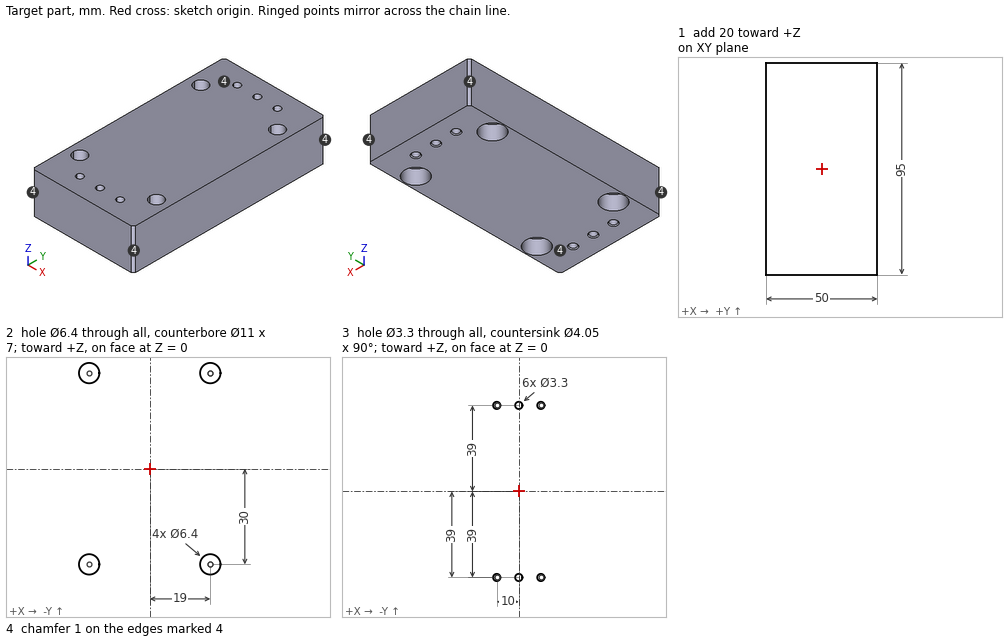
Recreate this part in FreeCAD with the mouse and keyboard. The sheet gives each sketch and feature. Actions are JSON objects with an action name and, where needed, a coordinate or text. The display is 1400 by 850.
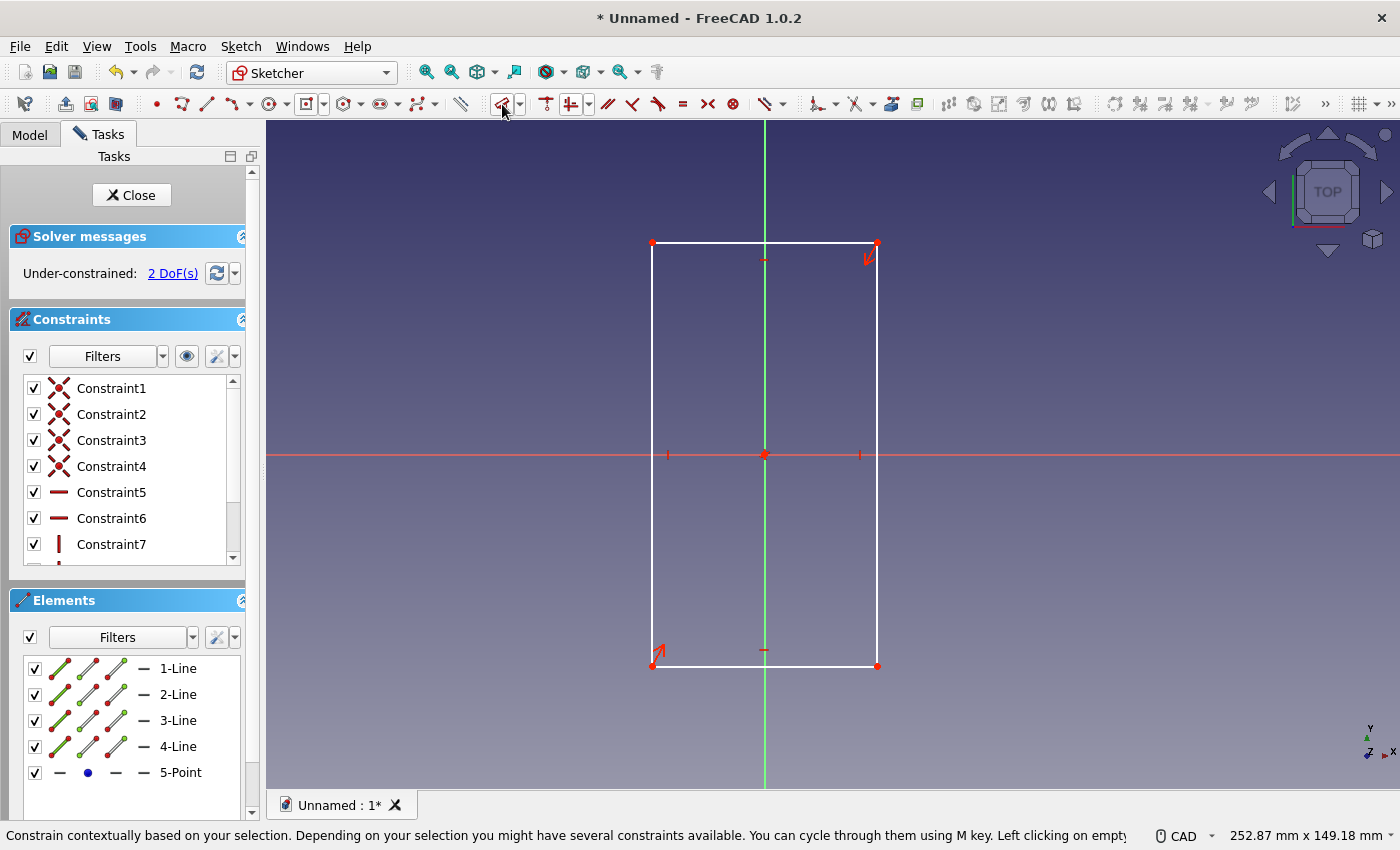
{"action": "left_click", "coordinate": [720, 667]}
{"action": "left_click", "coordinate": [713, 701]}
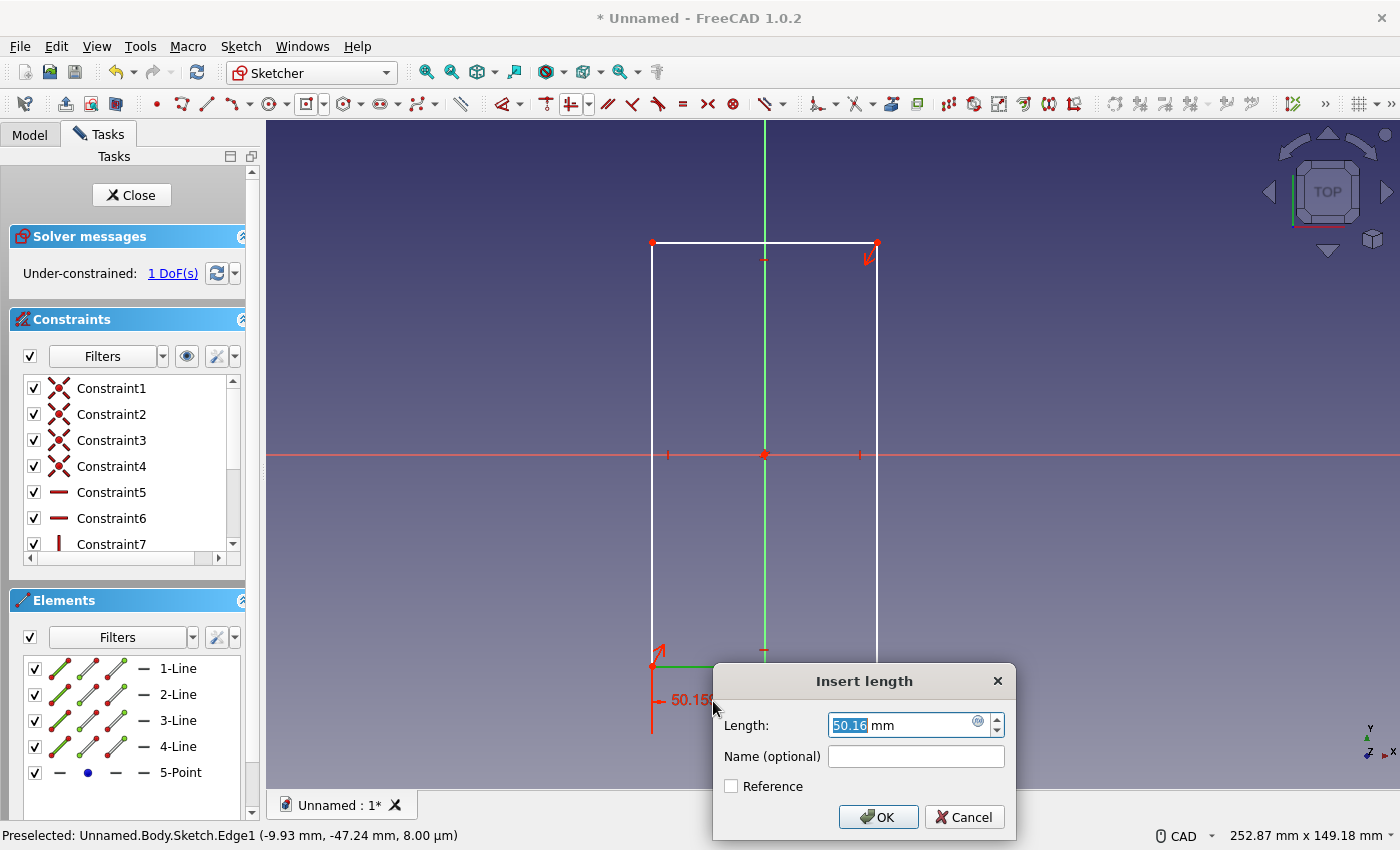
{"action": "type", "text": "50"}
{"action": "key", "text": "Return"}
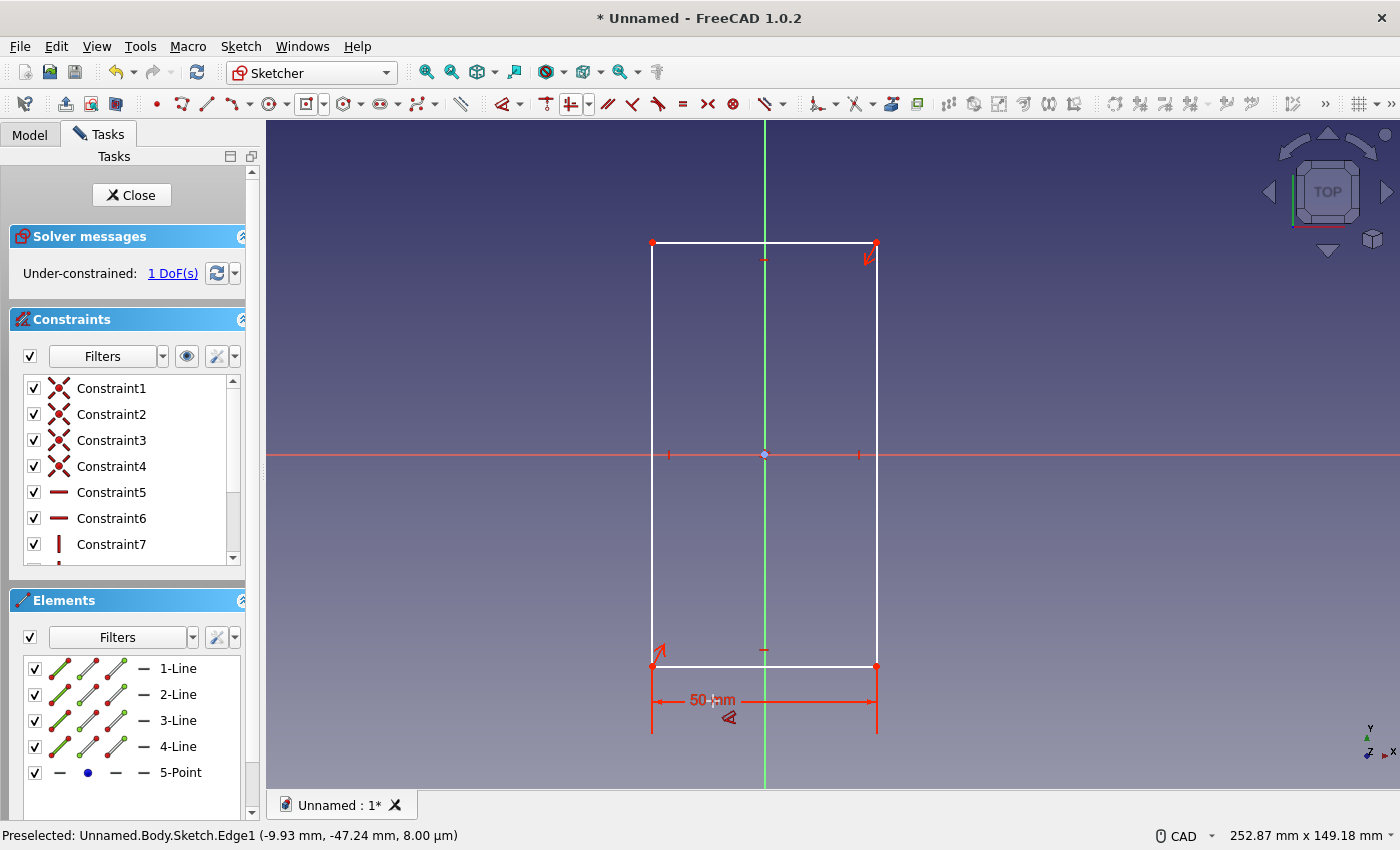
{"action": "left_click", "coordinate": [877, 540]}
{"action": "left_click", "coordinate": [911, 357]}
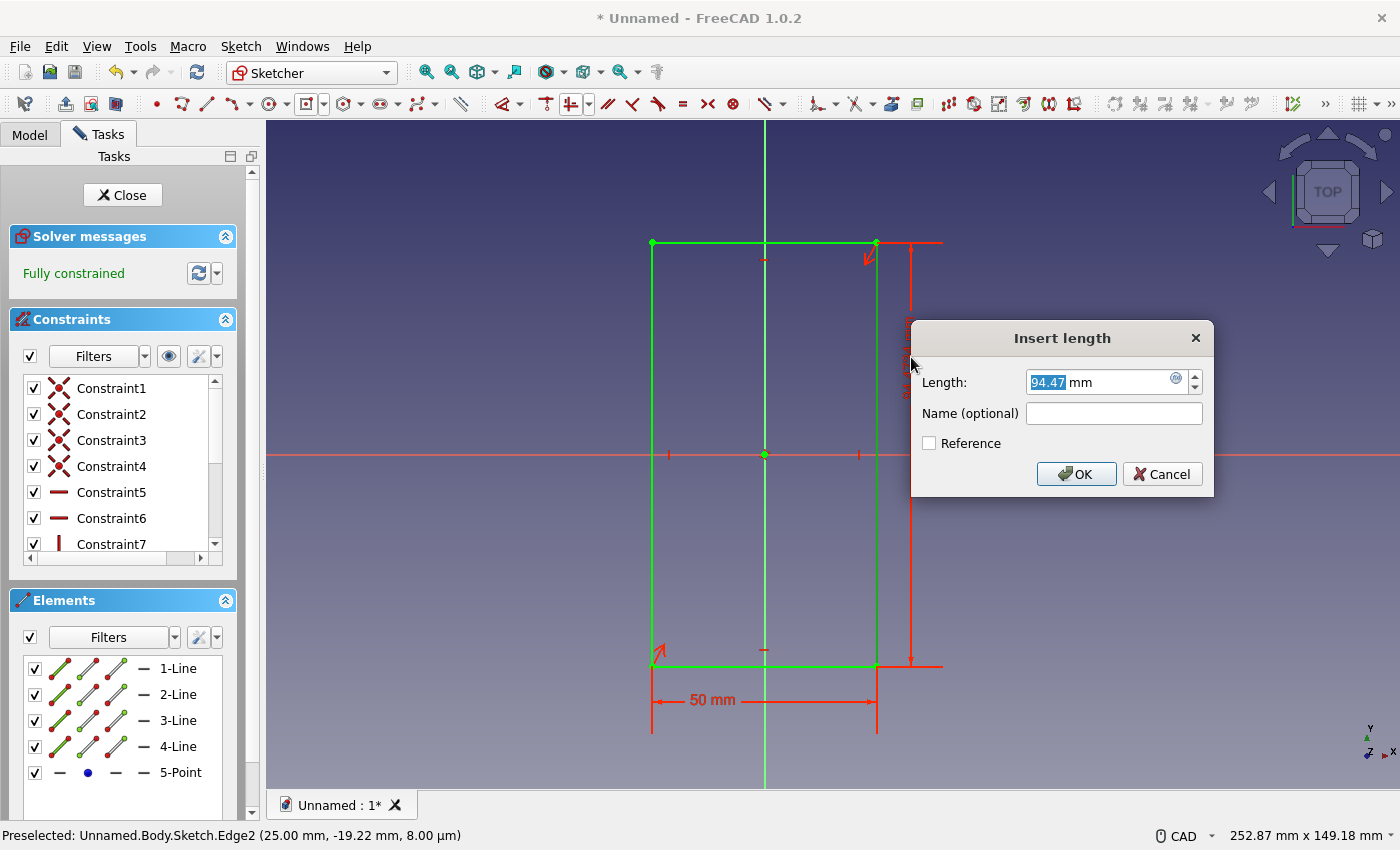
{"action": "type", "text": "95"}
{"action": "key", "text": "Return"}
{"action": "key", "text": "Escape"}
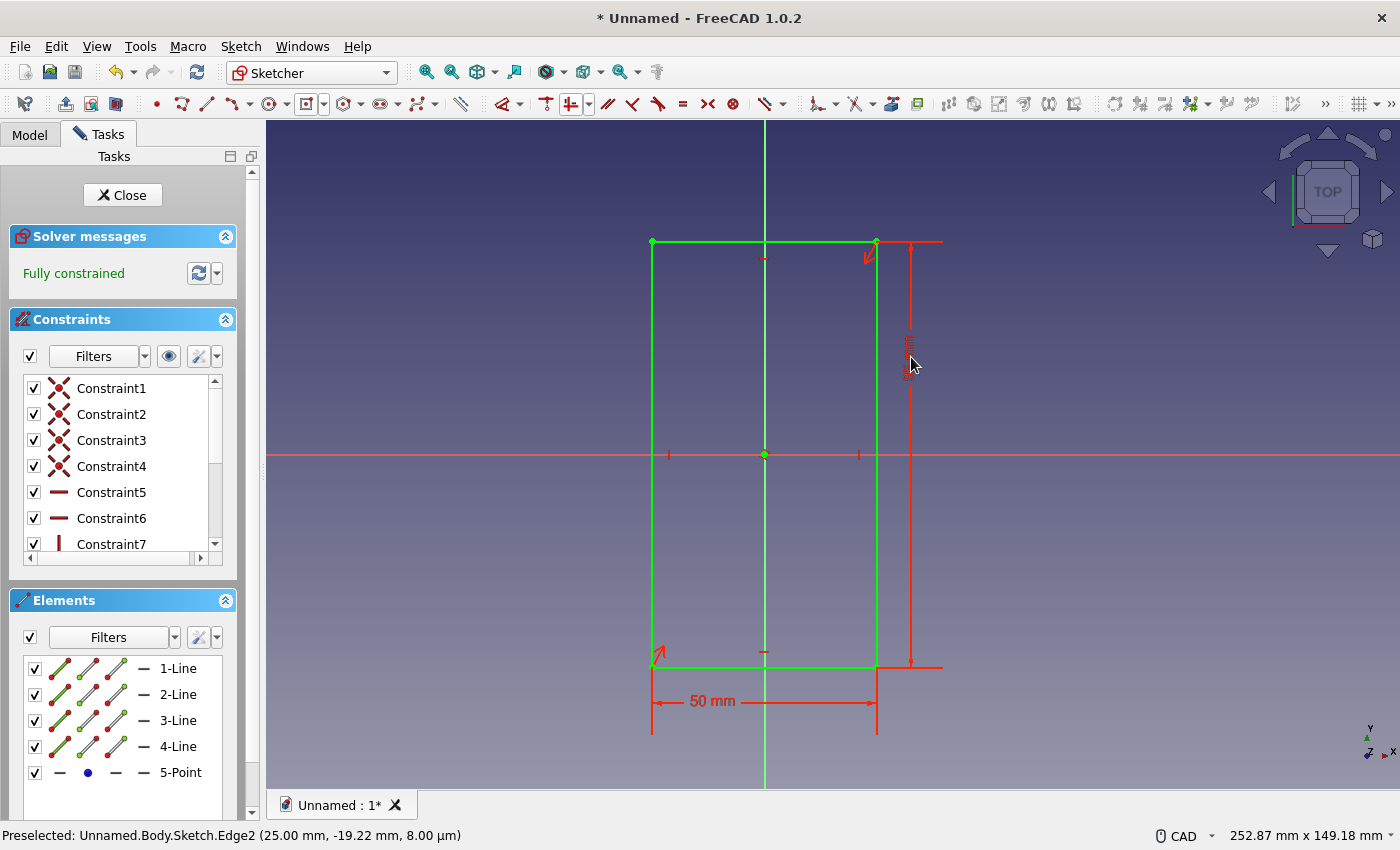
{"action": "left_click", "coordinate": [123, 195]}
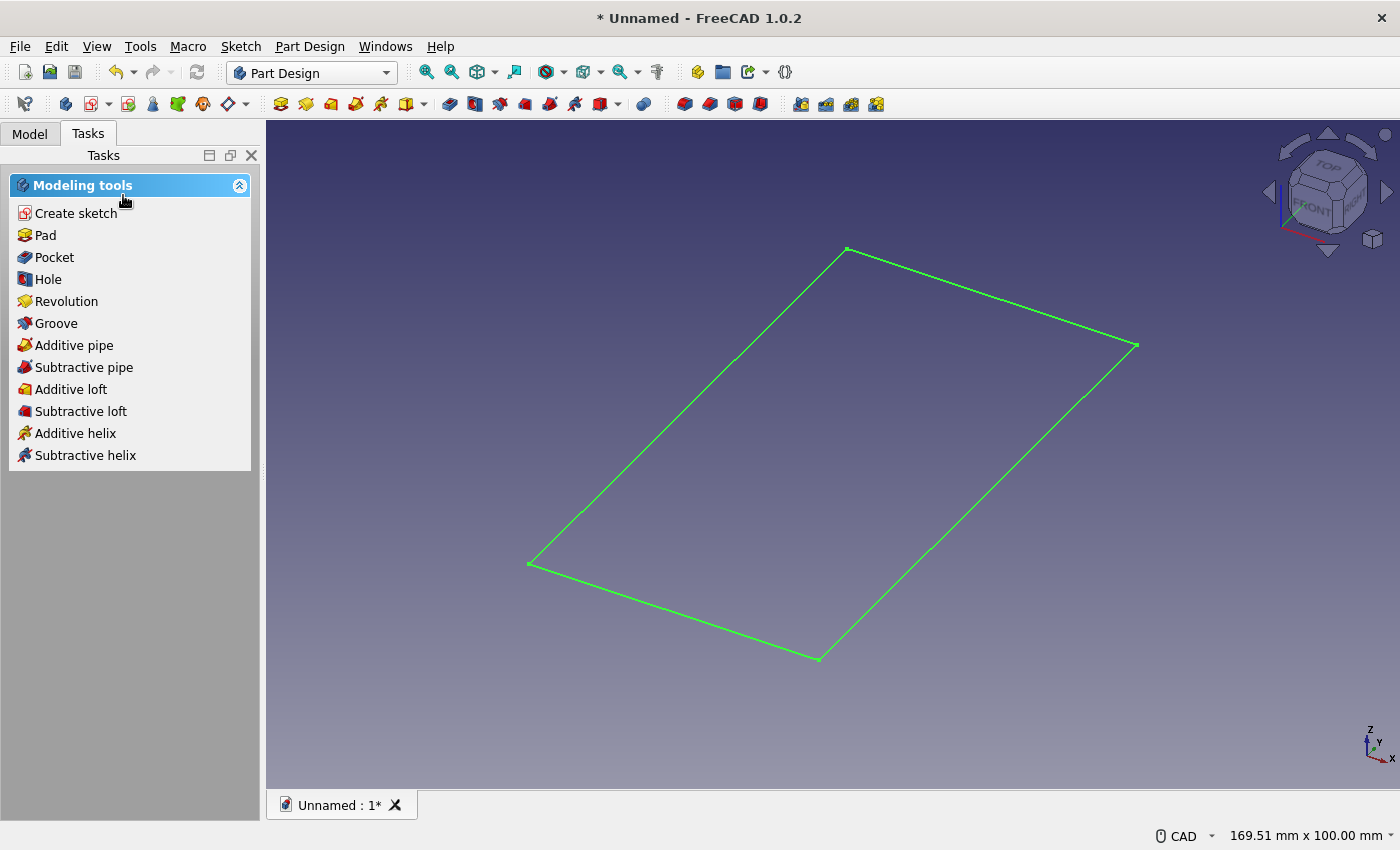
{"action": "left_click", "coordinate": [281, 104]}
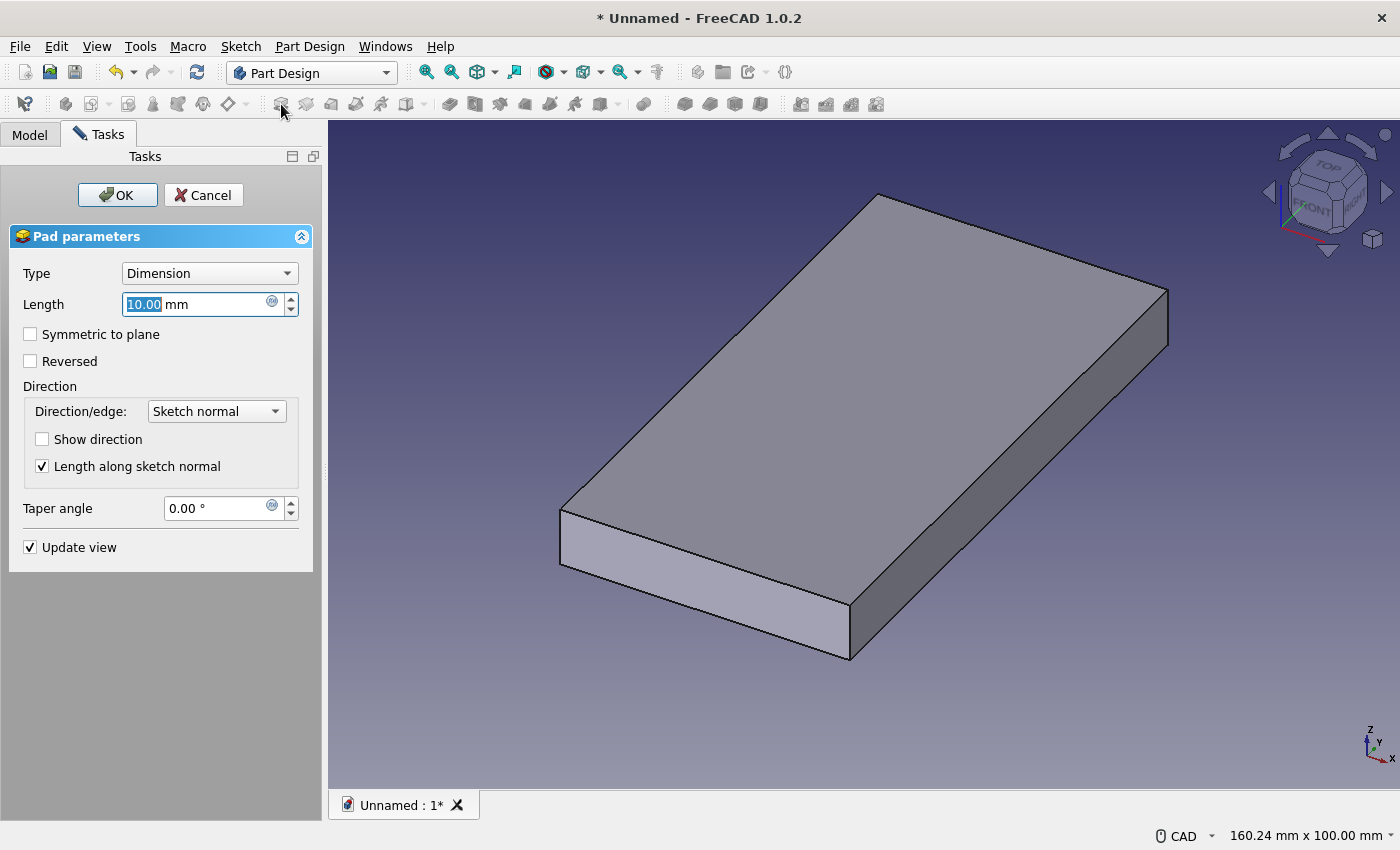
{"action": "type", "text": "20"}
{"action": "key", "text": "Tab"}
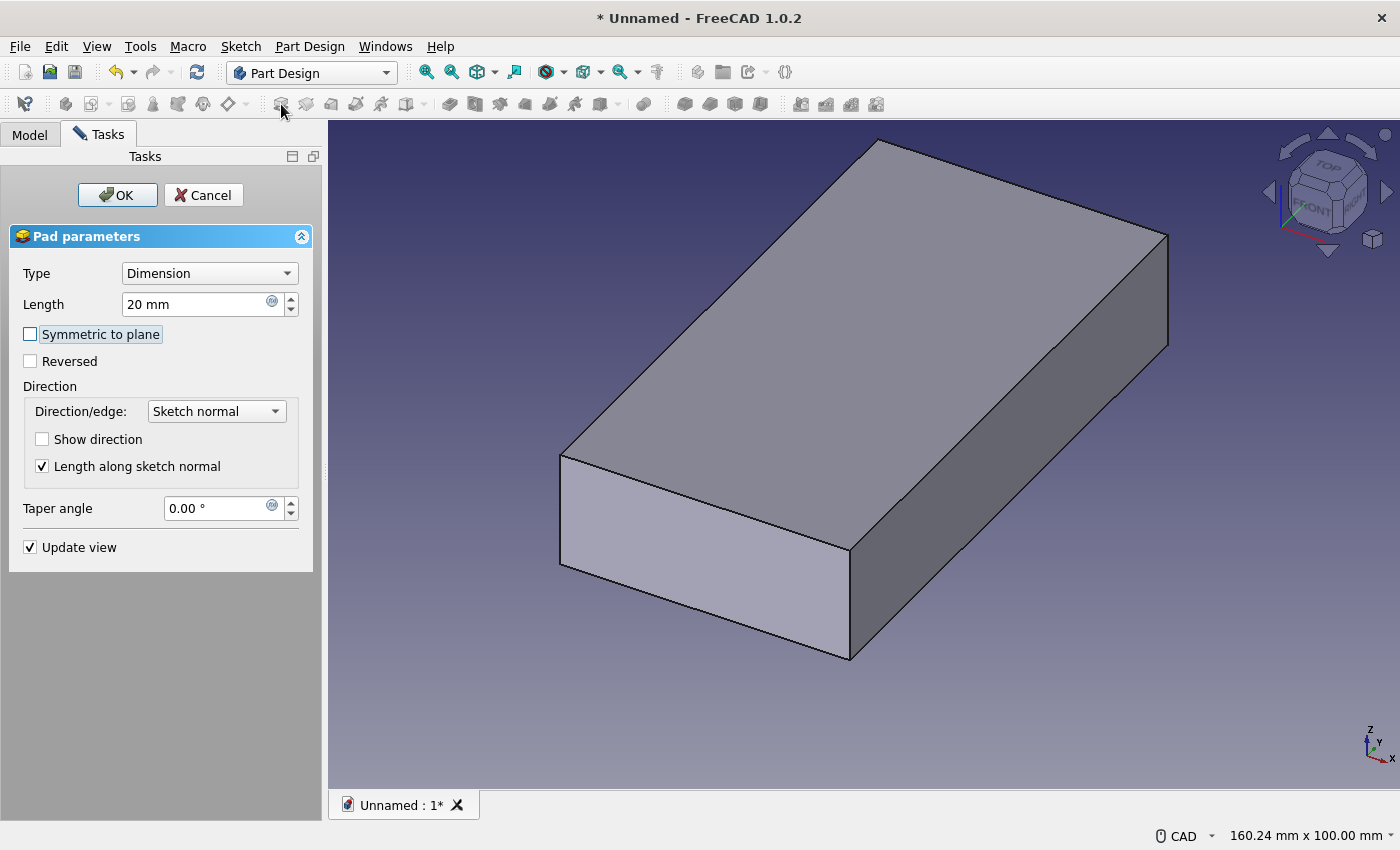
{"action": "left_click", "coordinate": [118, 195]}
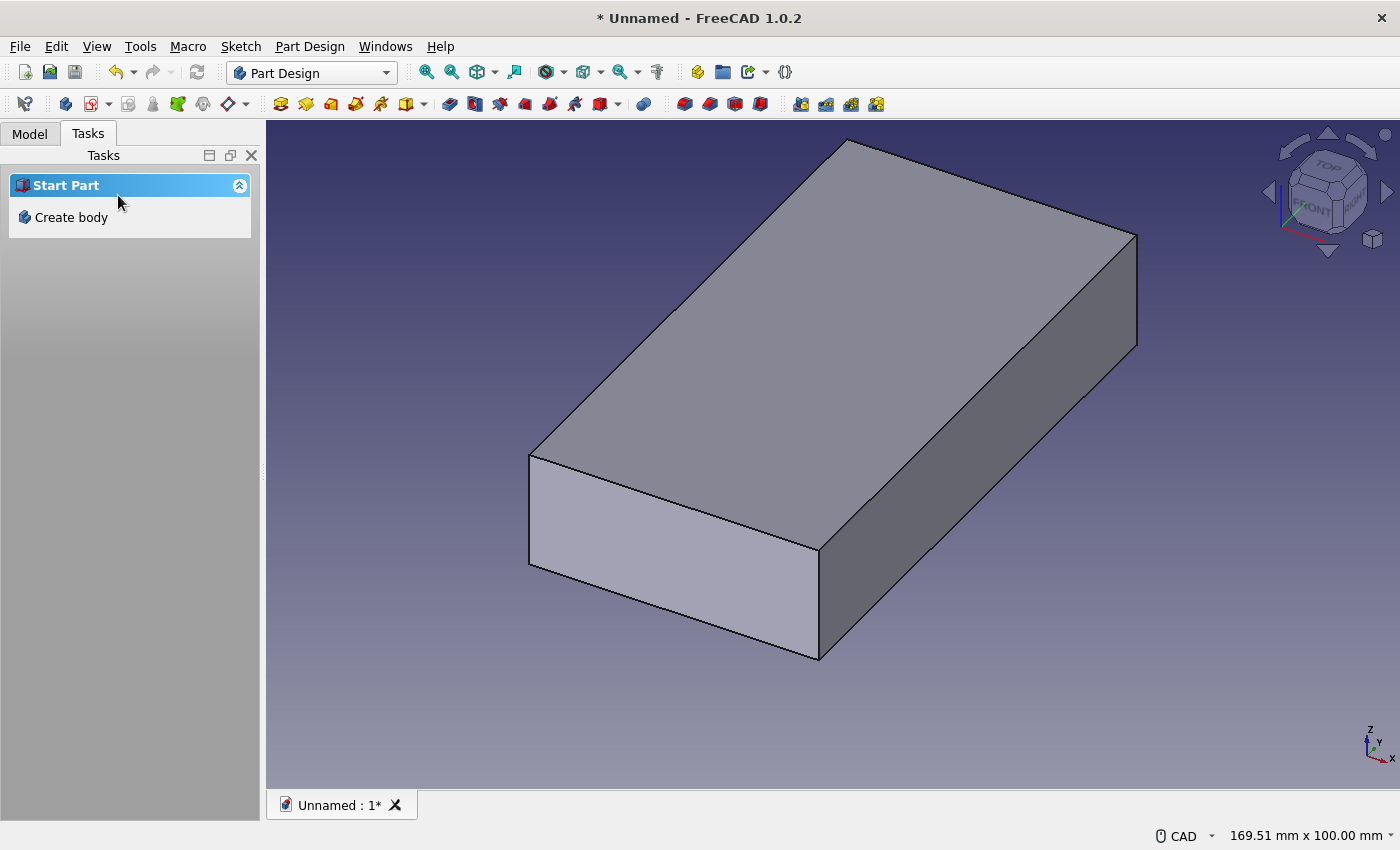
{"action": "key", "text": "5"}